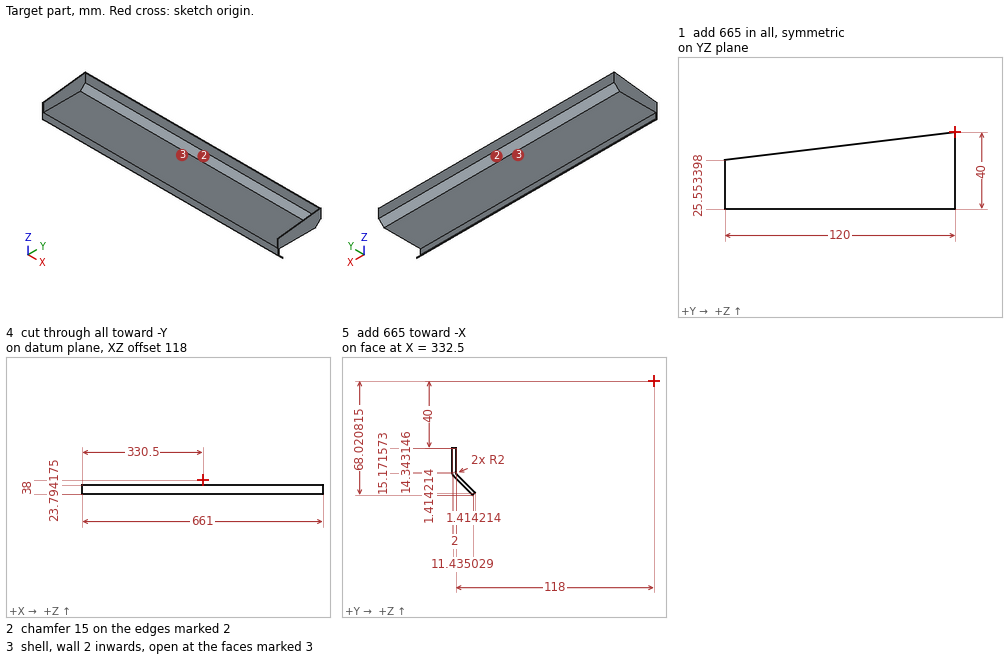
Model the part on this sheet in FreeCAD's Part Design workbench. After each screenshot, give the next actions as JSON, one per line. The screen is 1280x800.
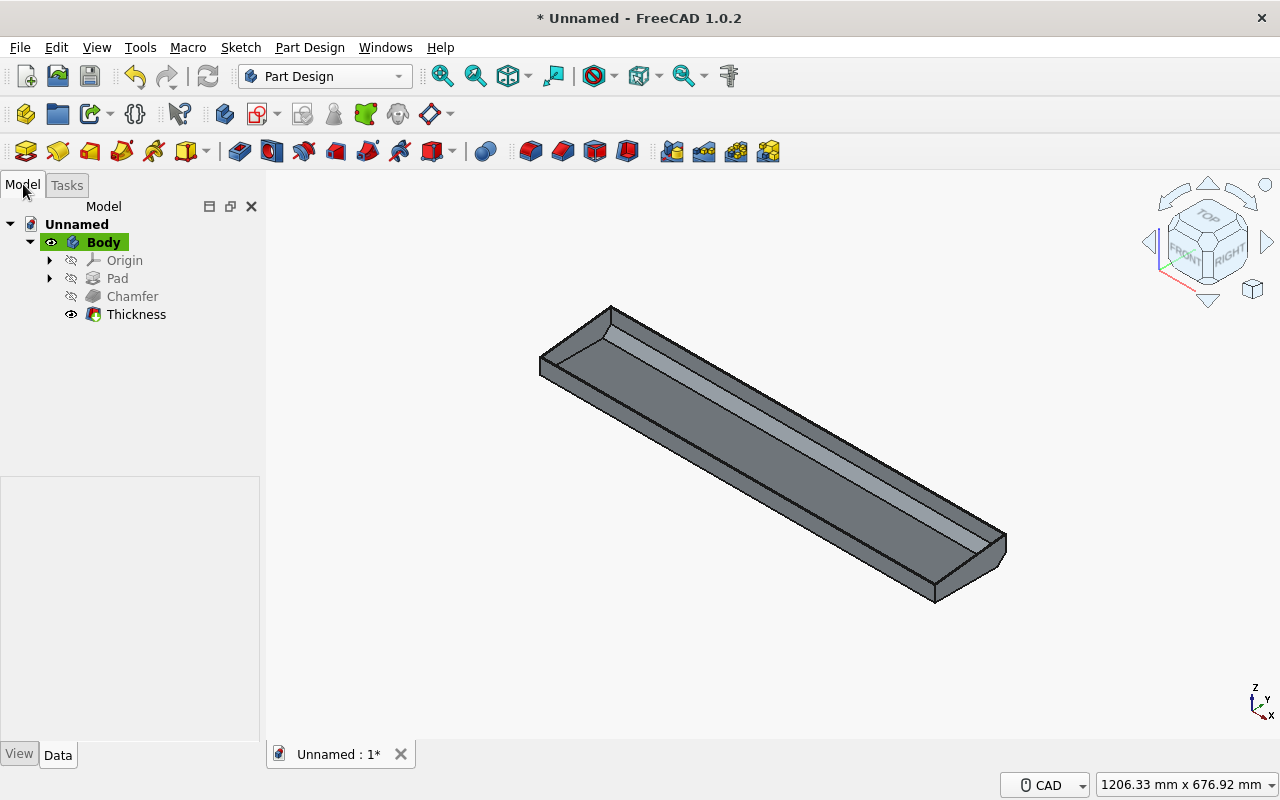
{"action": "left_click", "coordinate": [50, 260]}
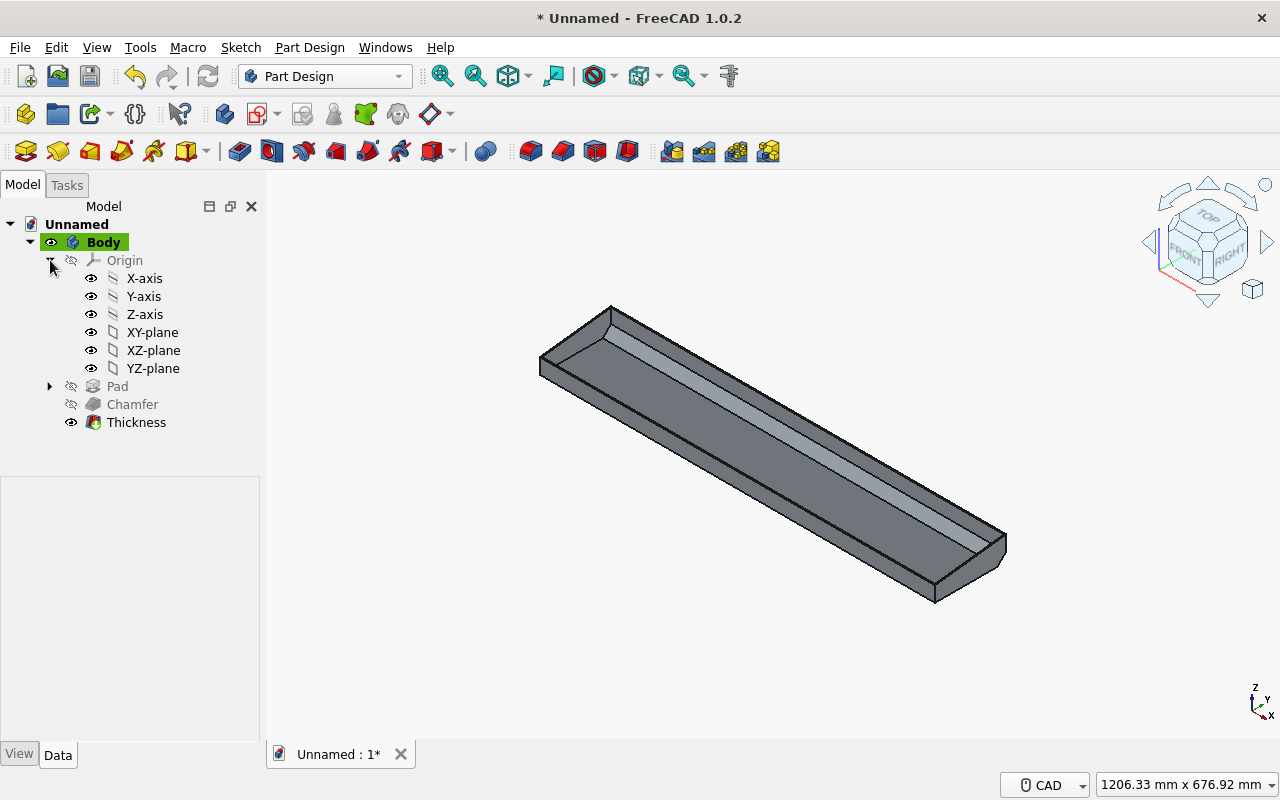
{"action": "left_click", "coordinate": [136, 350]}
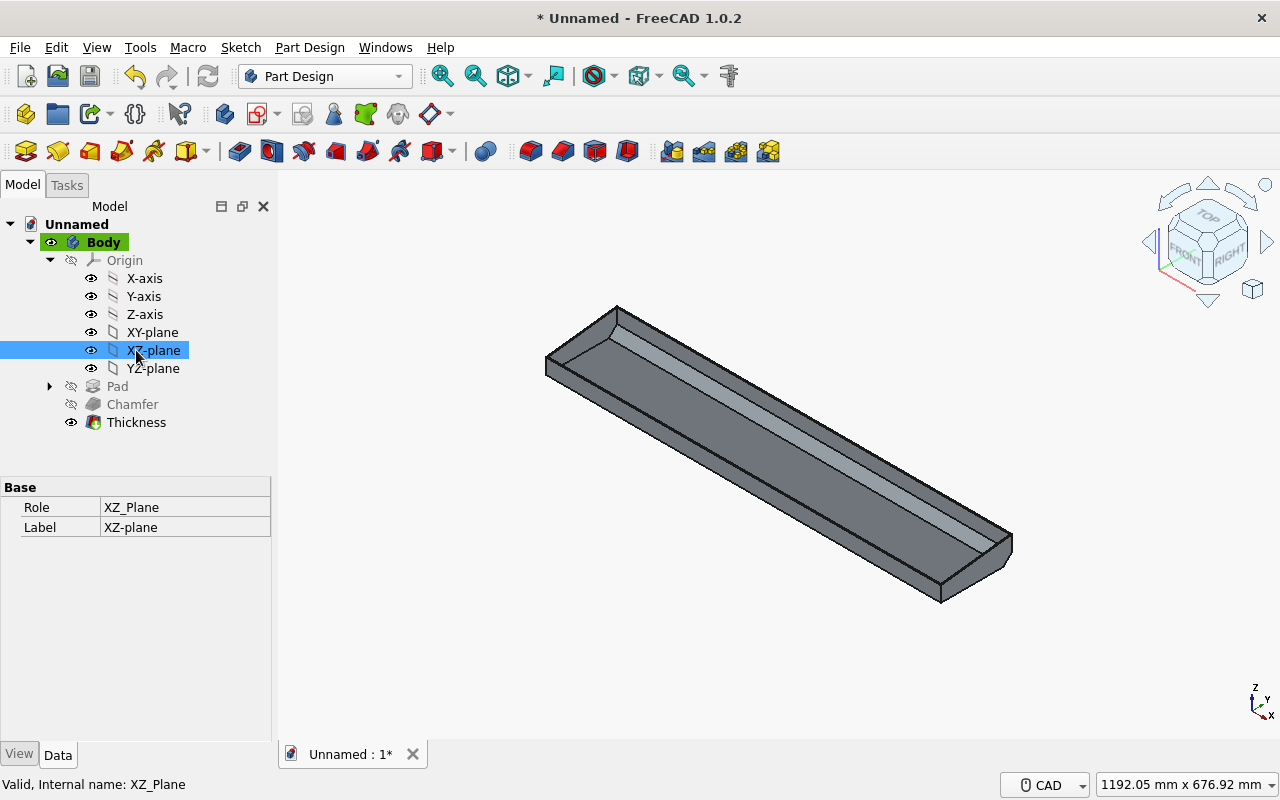
{"action": "left_click", "coordinate": [430, 114]}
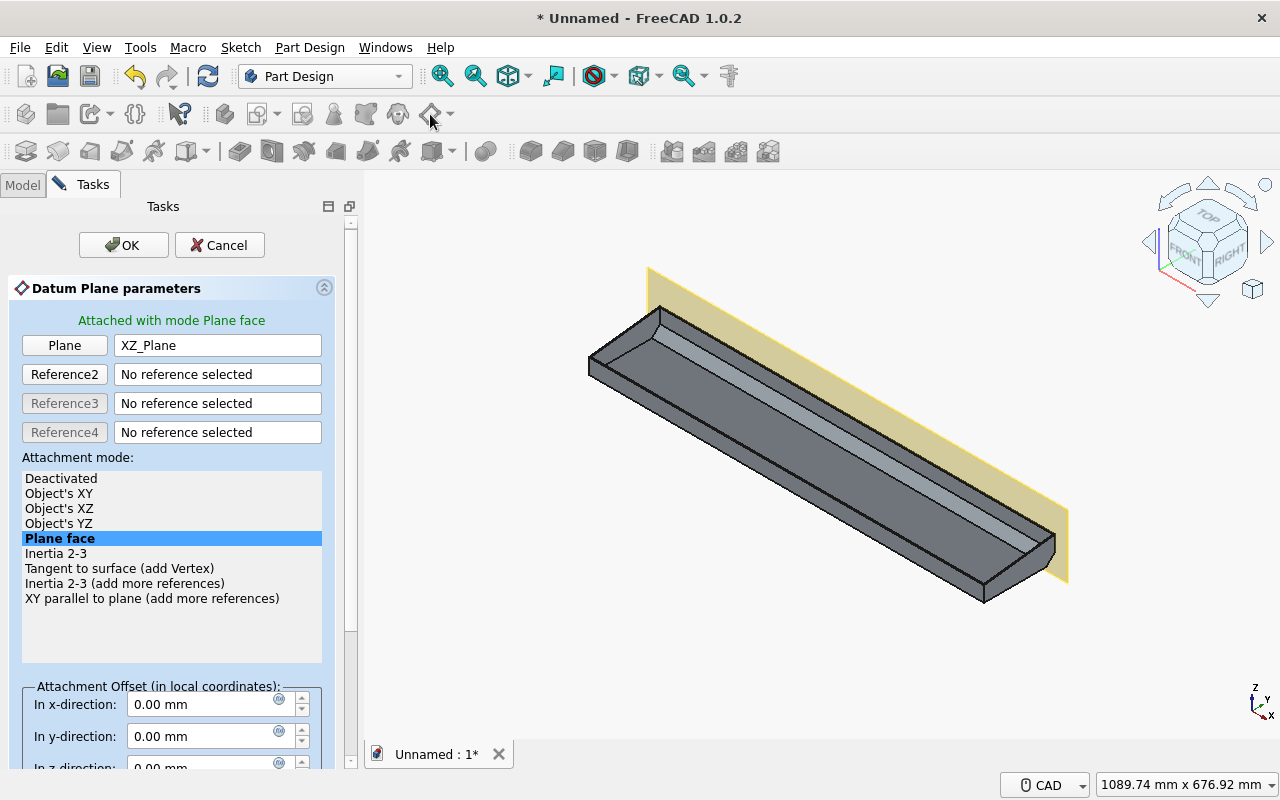
{"action": "scroll", "coordinate": [351, 492], "scroll_direction": "down", "scroll_amount": 2}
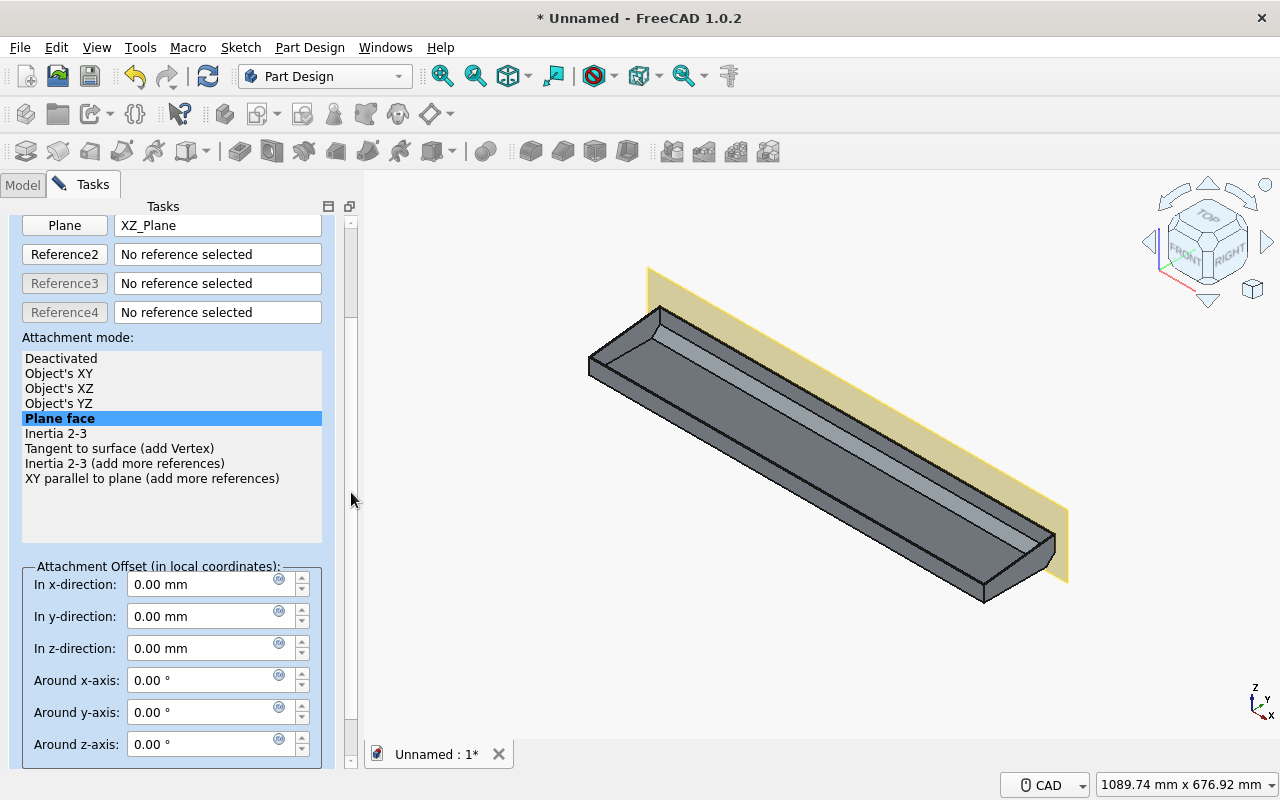
{"action": "triple_click", "coordinate": [210, 648]}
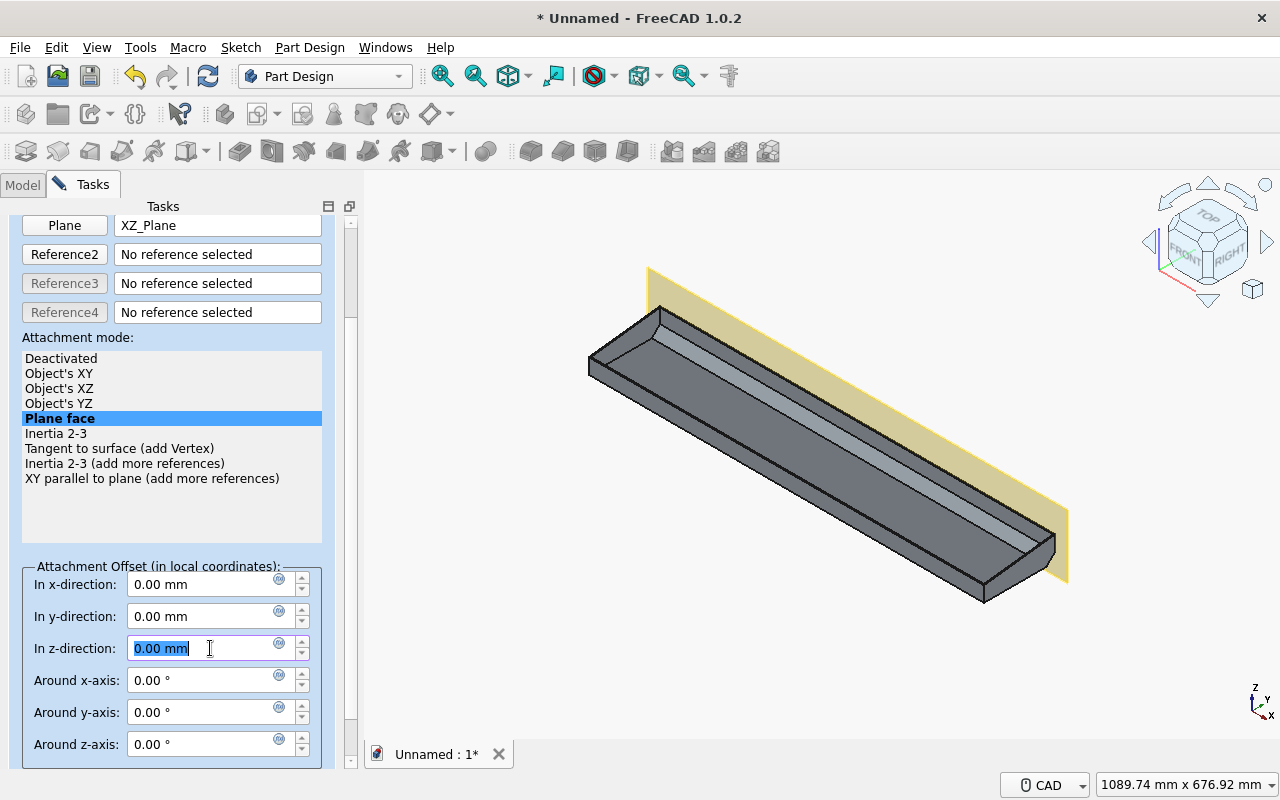
{"action": "type", "text": "118"}
{"action": "key", "text": "Tab"}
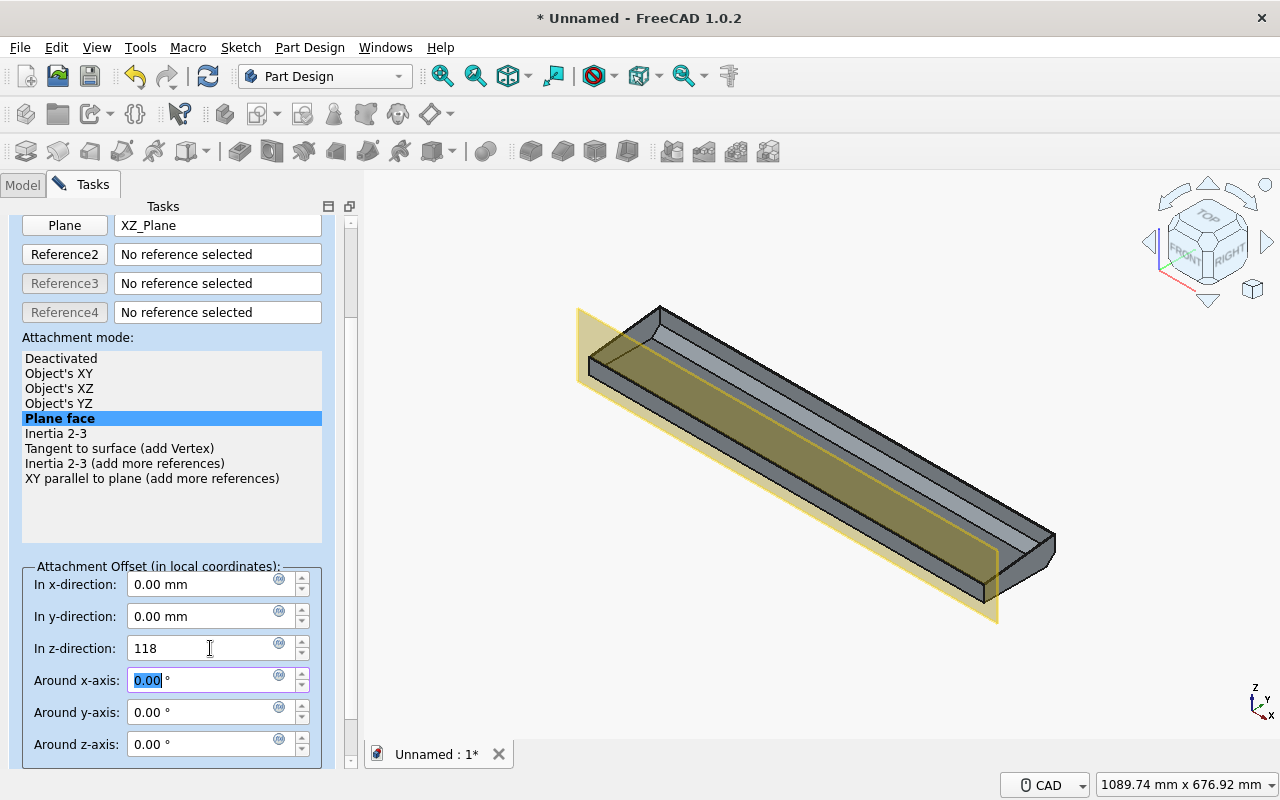
{"action": "scroll", "coordinate": [351, 492], "scroll_direction": "up", "scroll_amount": 3}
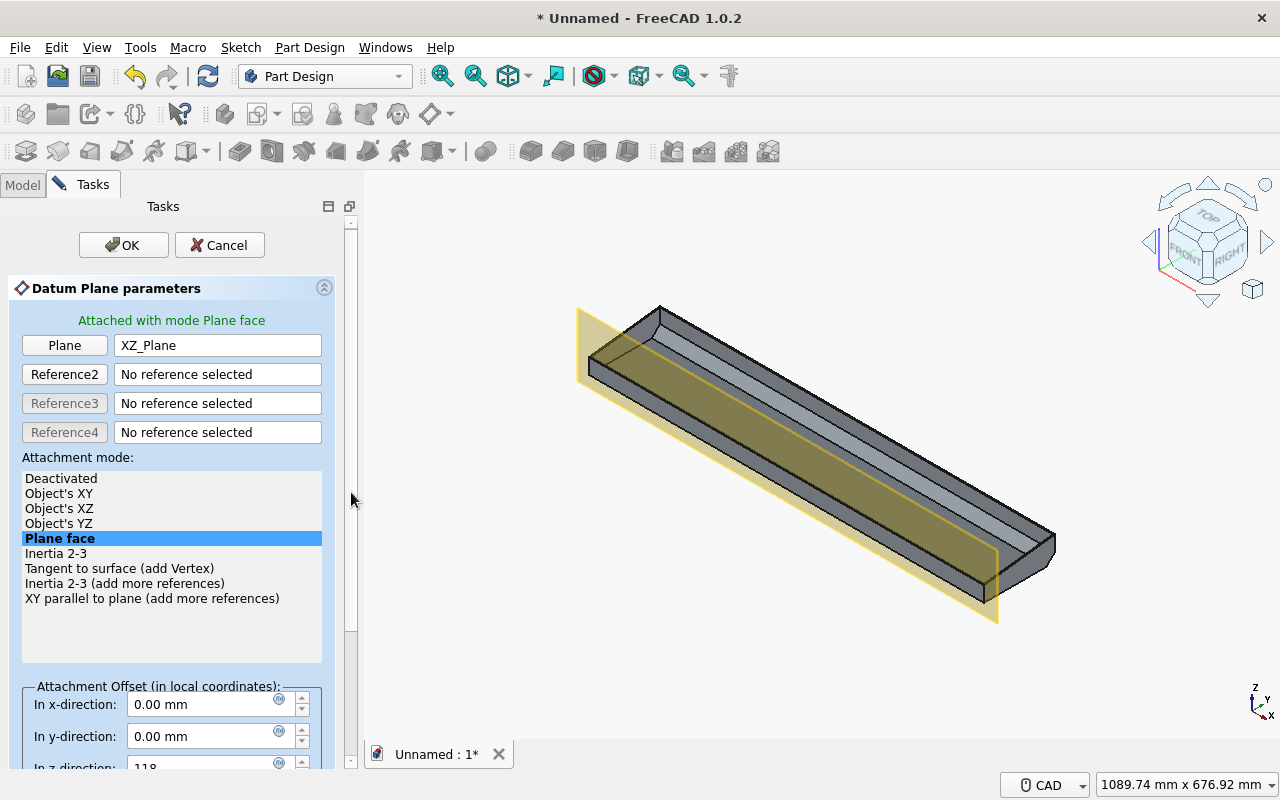
{"action": "left_click", "coordinate": [124, 245]}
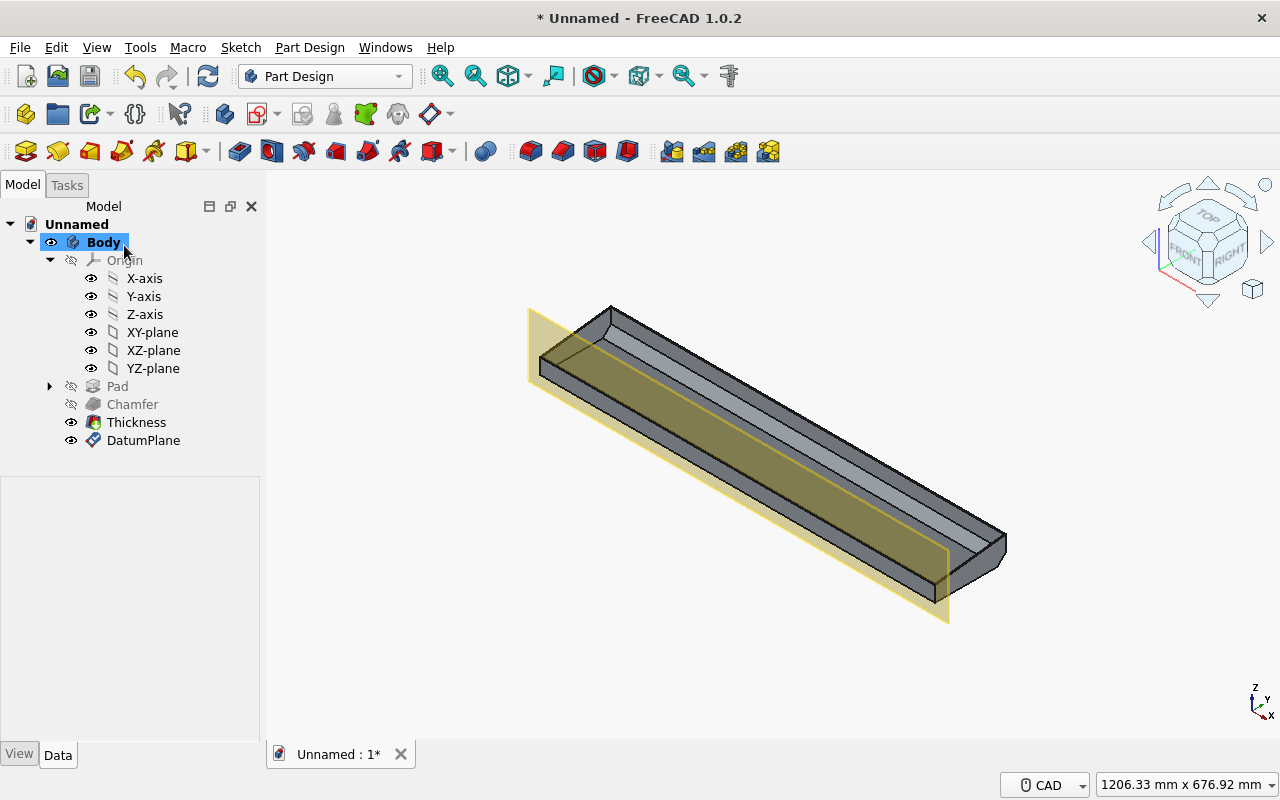
{"action": "left_click", "coordinate": [116, 440]}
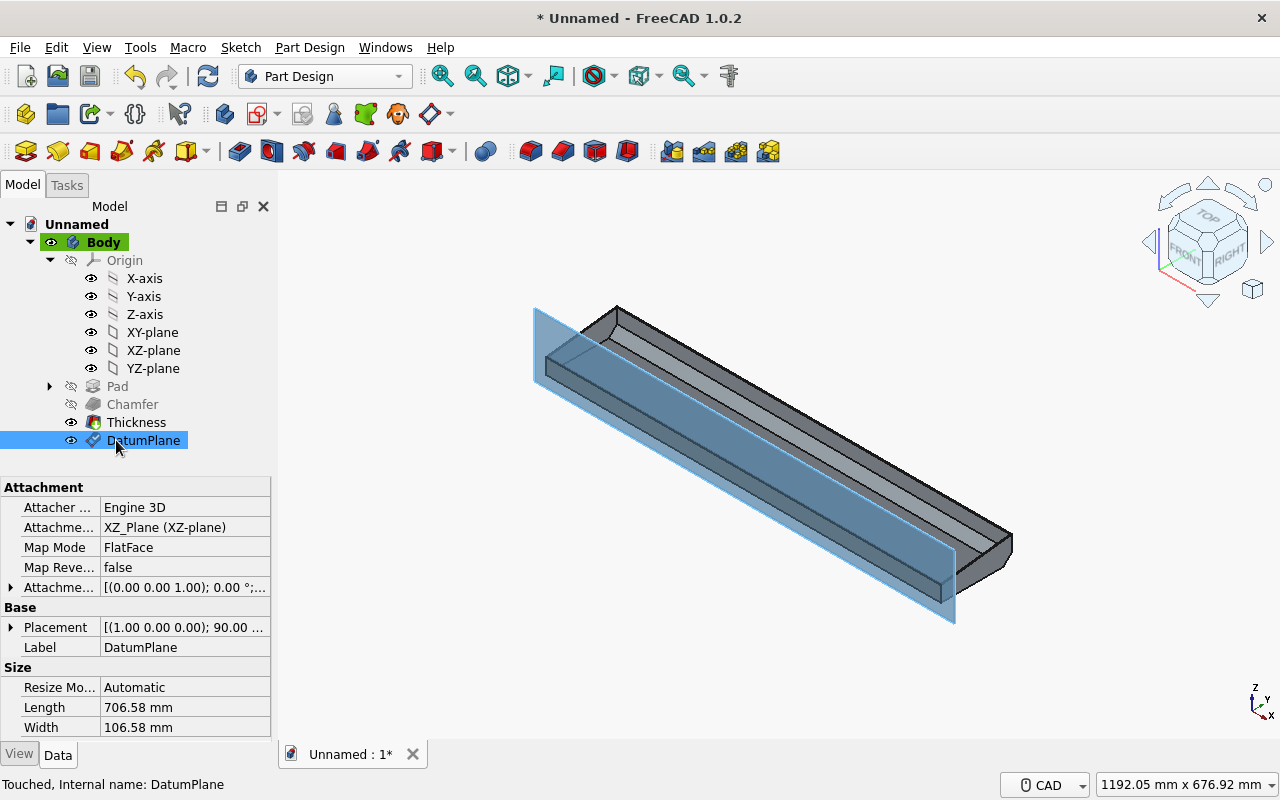
{"action": "left_click", "coordinate": [258, 114]}